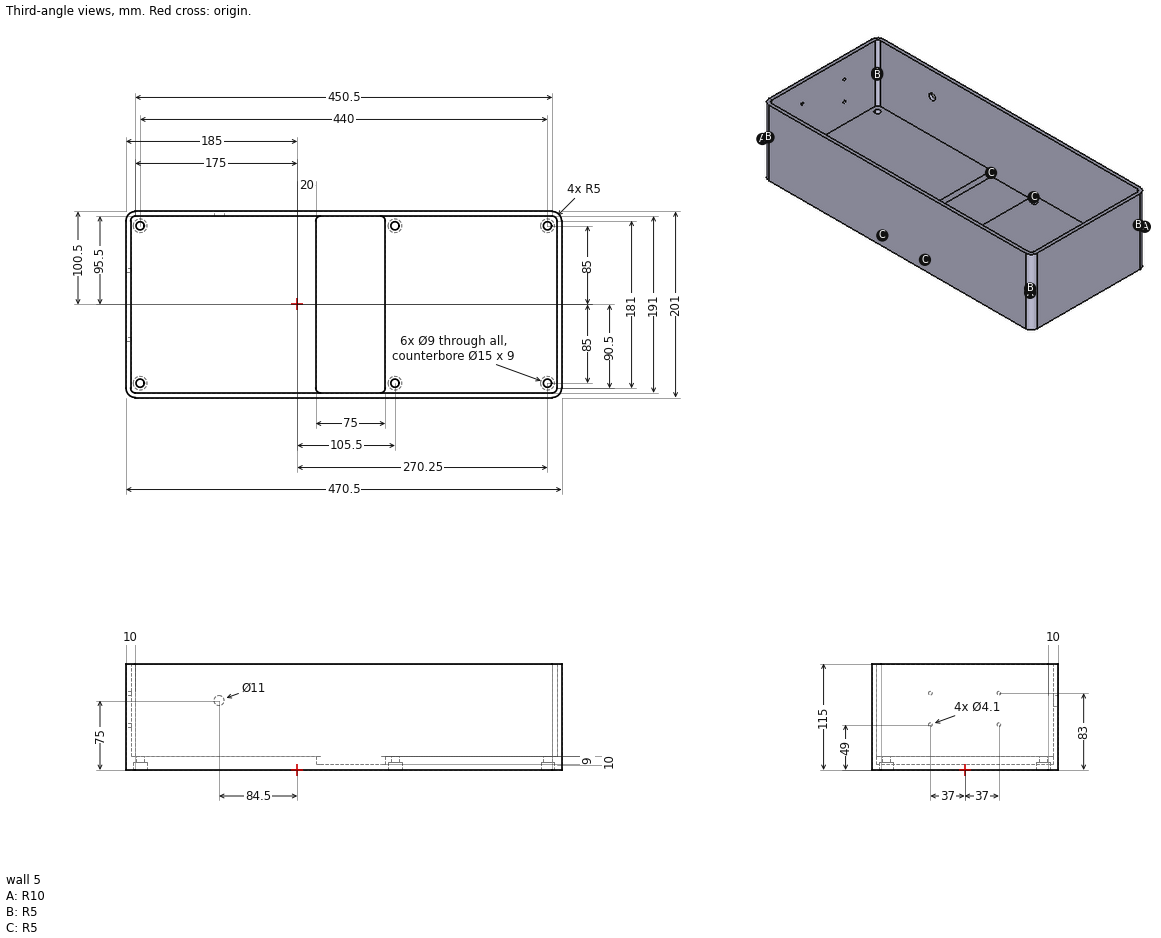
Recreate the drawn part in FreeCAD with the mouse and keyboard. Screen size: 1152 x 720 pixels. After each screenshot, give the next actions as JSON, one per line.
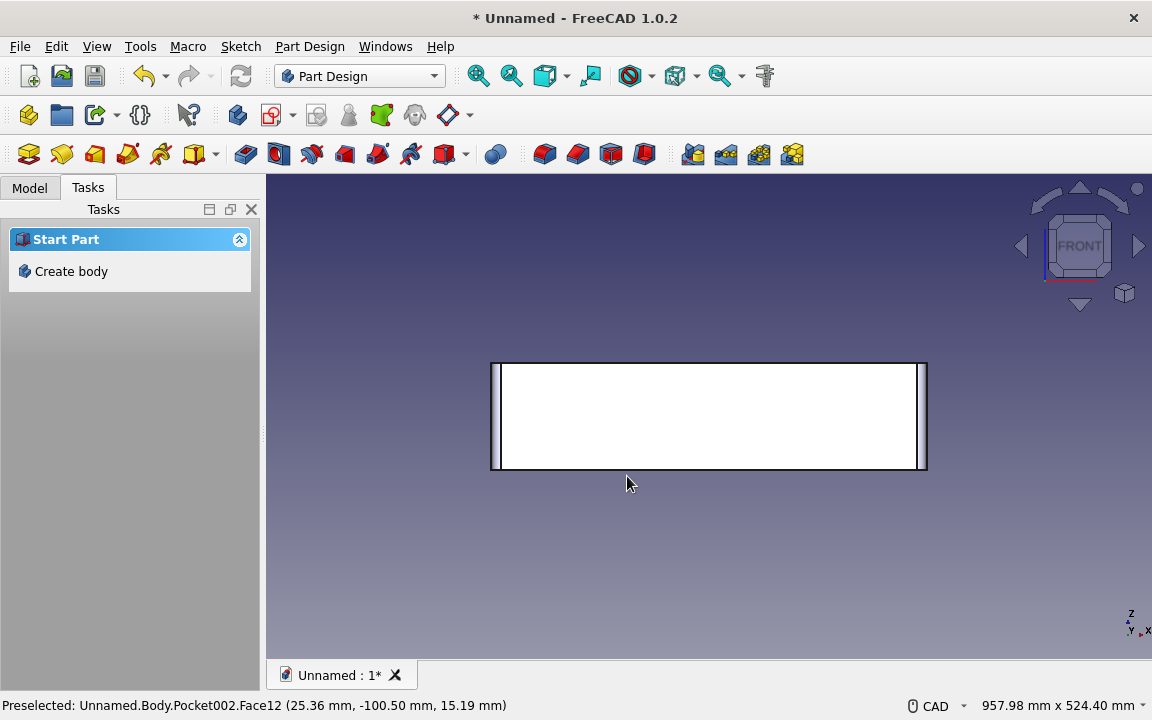
{"action": "scroll", "coordinate": [681, 459], "scroll_direction": "up", "scroll_amount": 8}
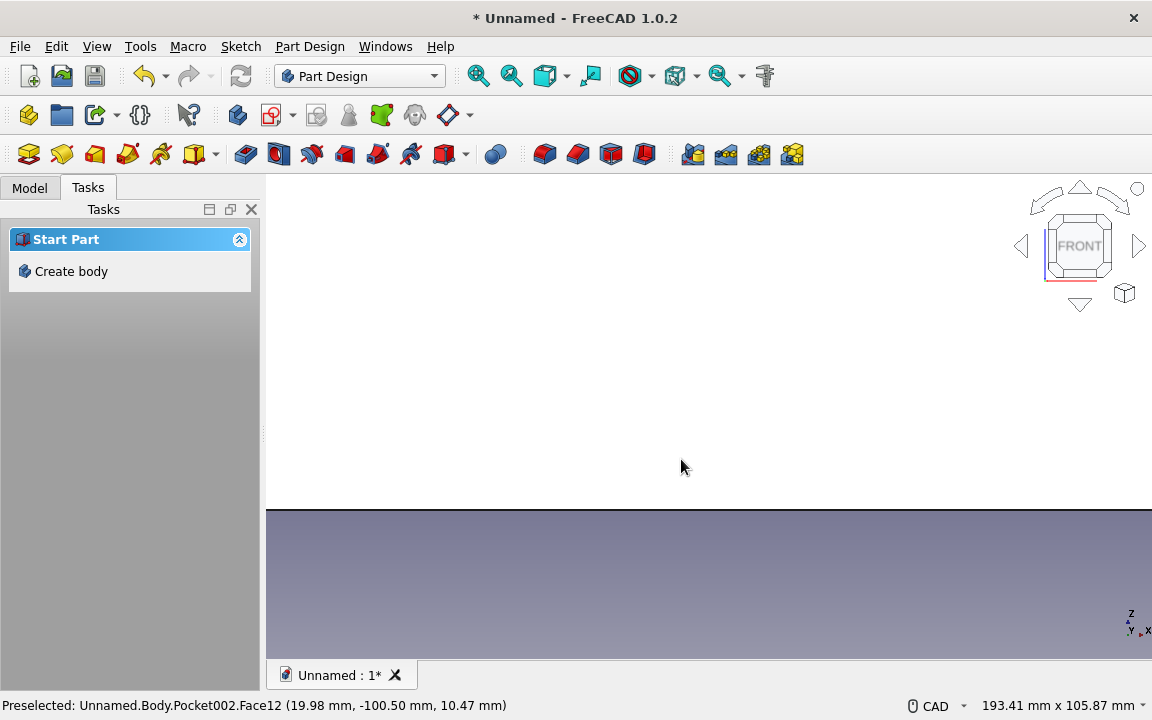
{"action": "key", "text": "v f"}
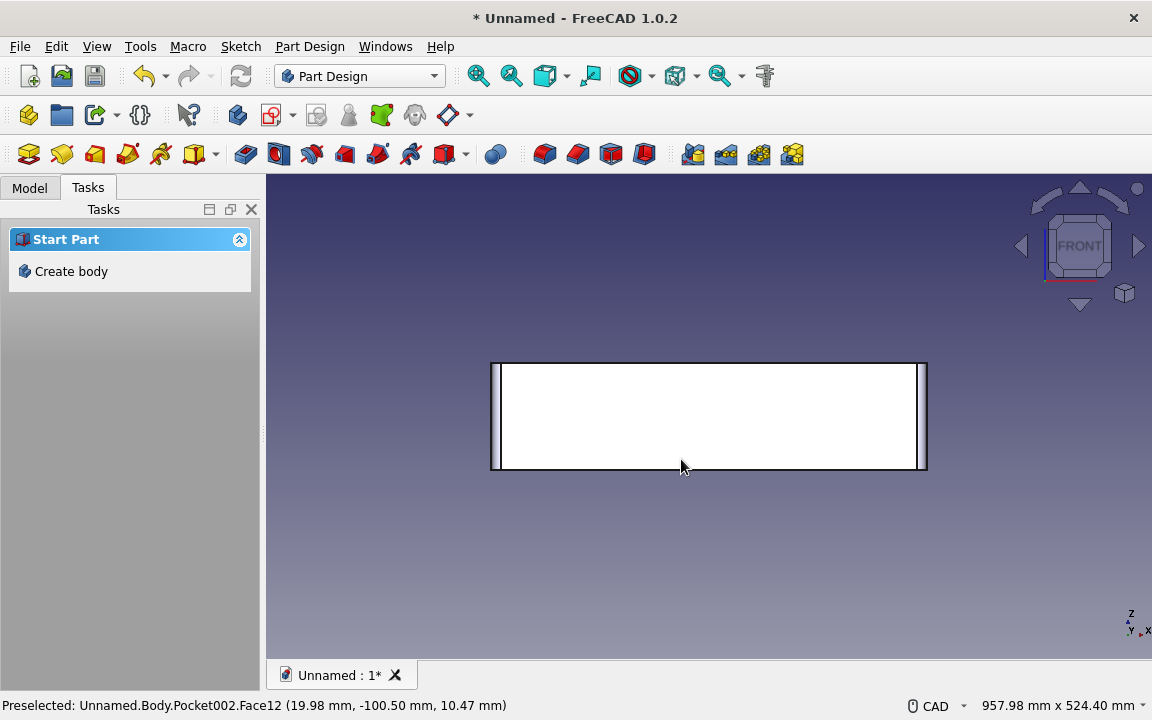
{"action": "key", "text": "3"}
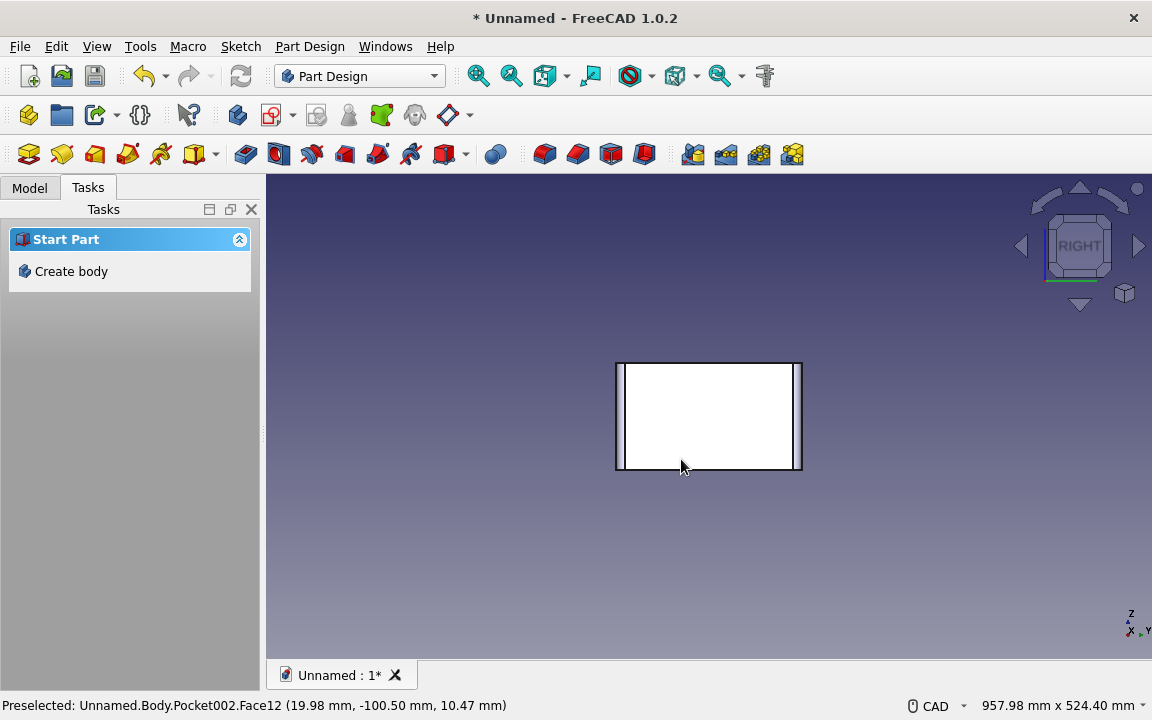
{"action": "key", "text": "v f"}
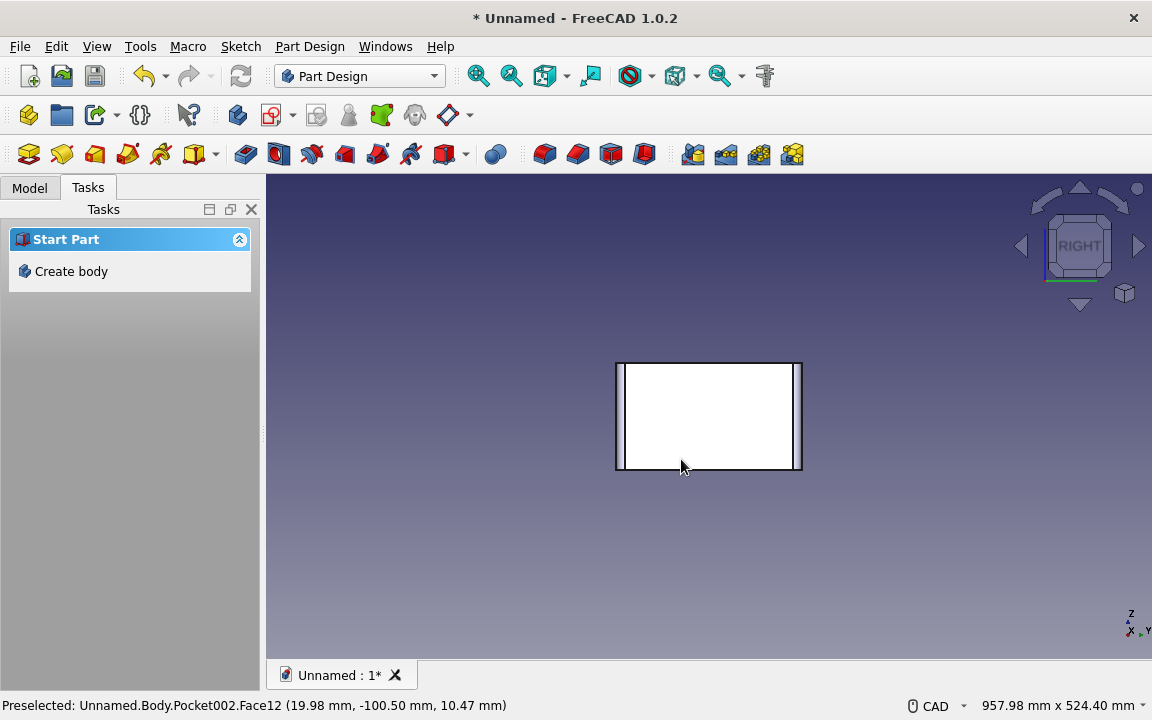
{"action": "scroll", "coordinate": [621, 459], "scroll_direction": "up", "scroll_amount": 8}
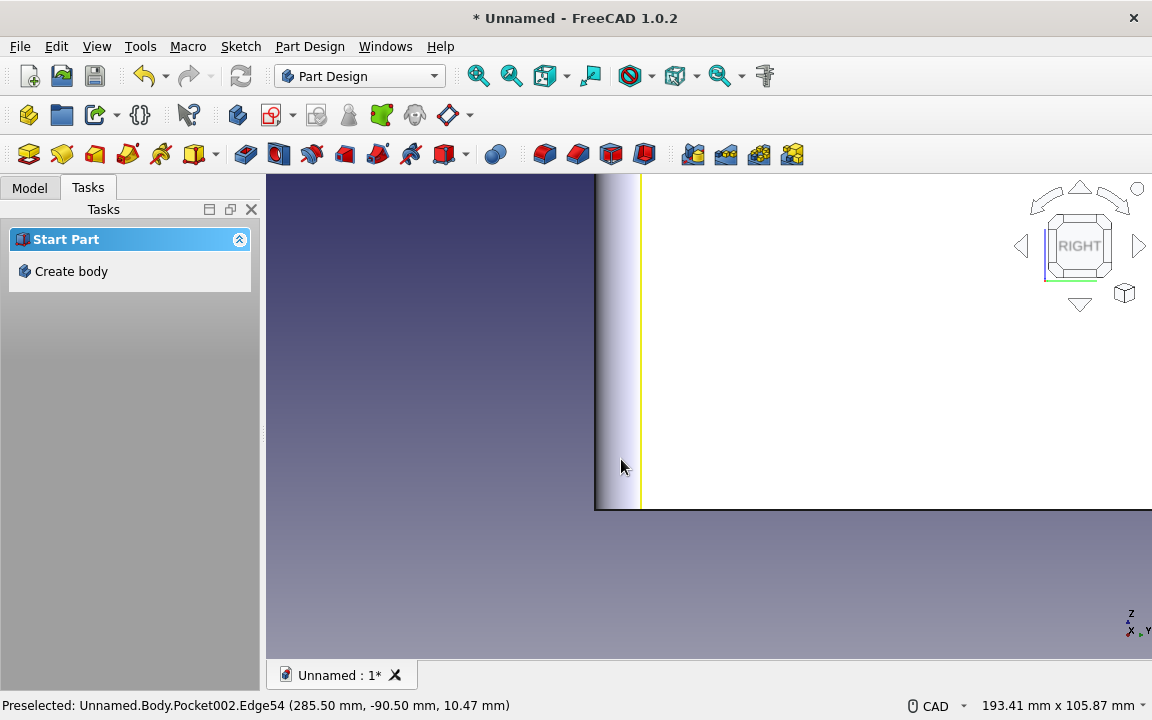
{"action": "key", "text": "v f"}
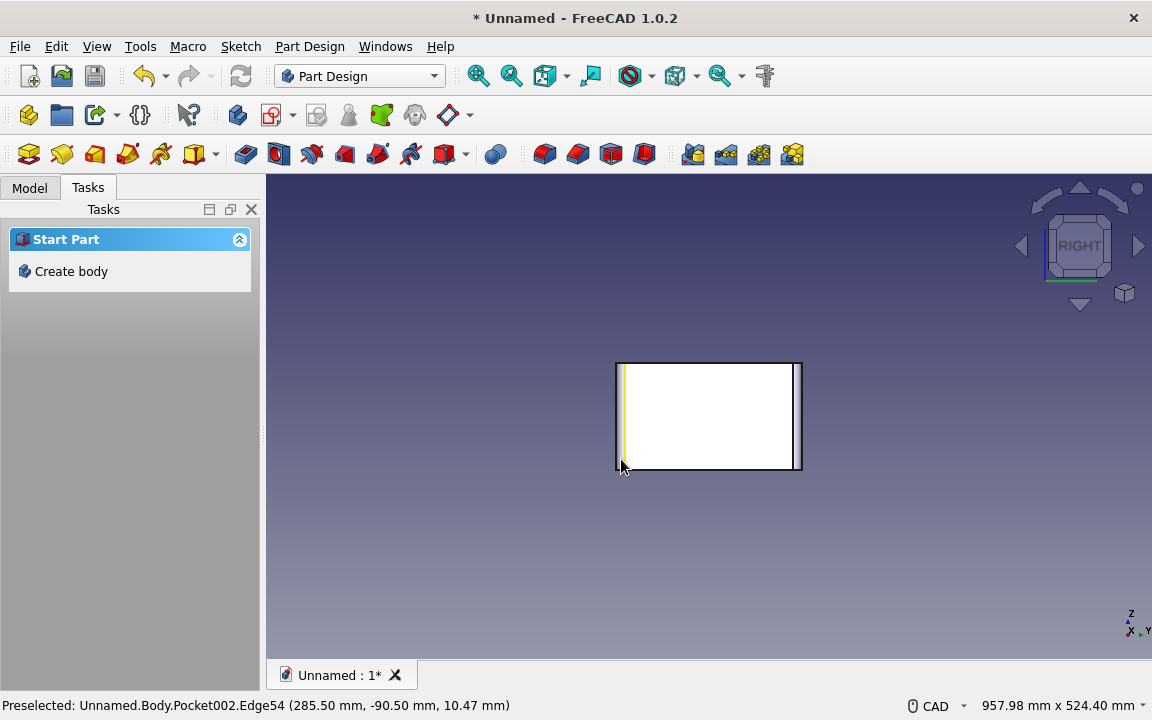
{"action": "key", "text": "5"}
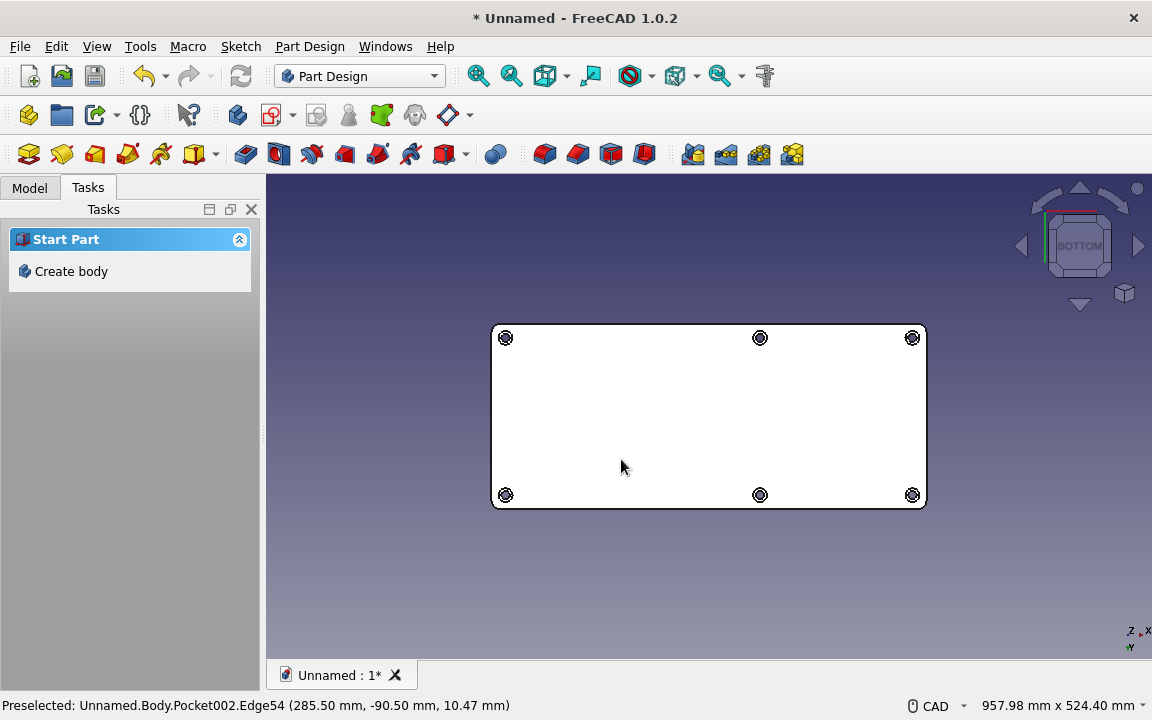
{"action": "scroll", "coordinate": [681, 327], "scroll_direction": "up", "scroll_amount": 8}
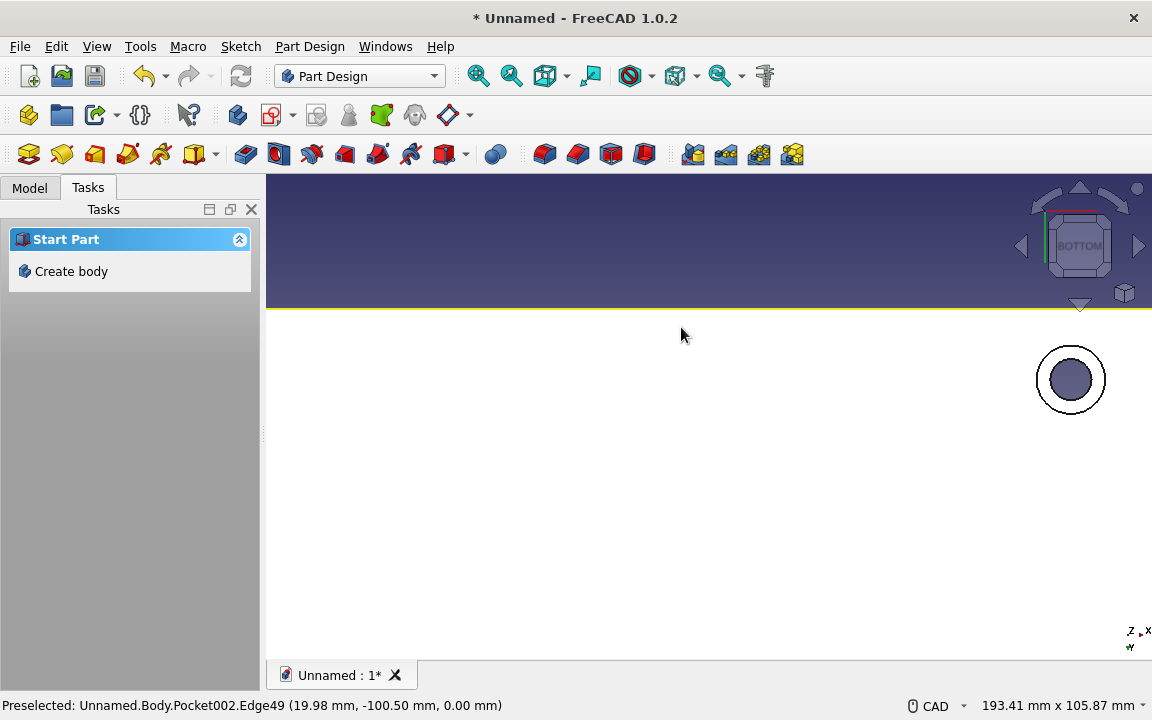
{"action": "left_click", "coordinate": [479, 76]}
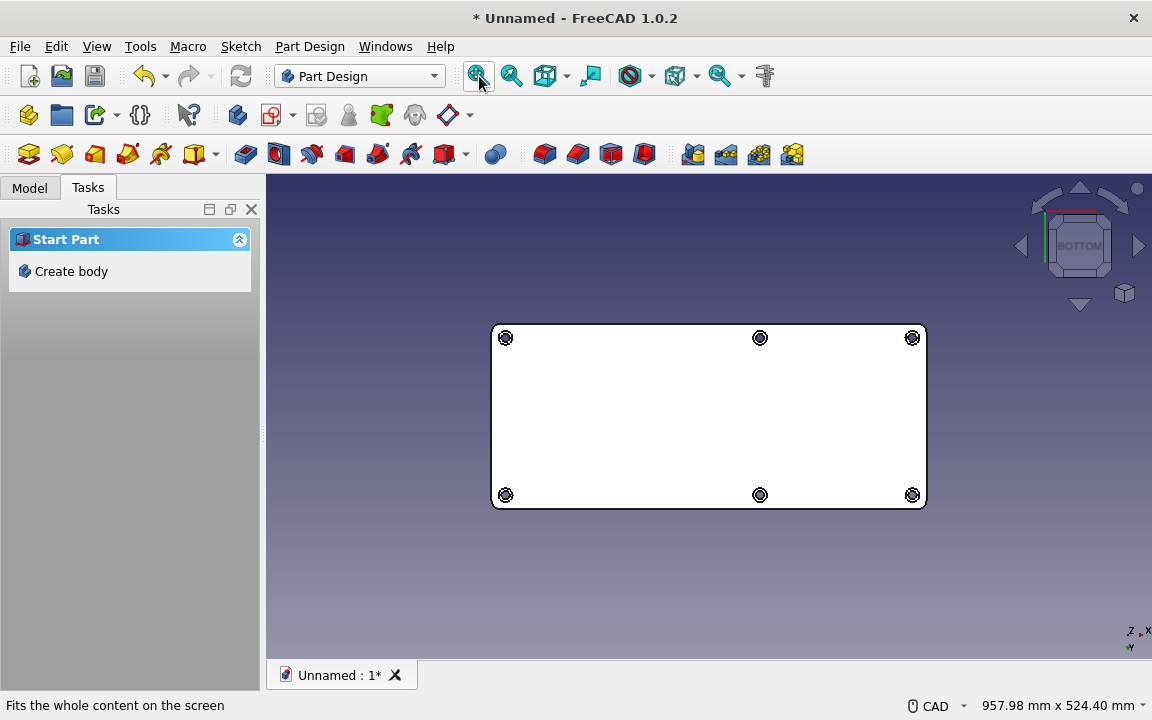
{"action": "key", "text": "4"}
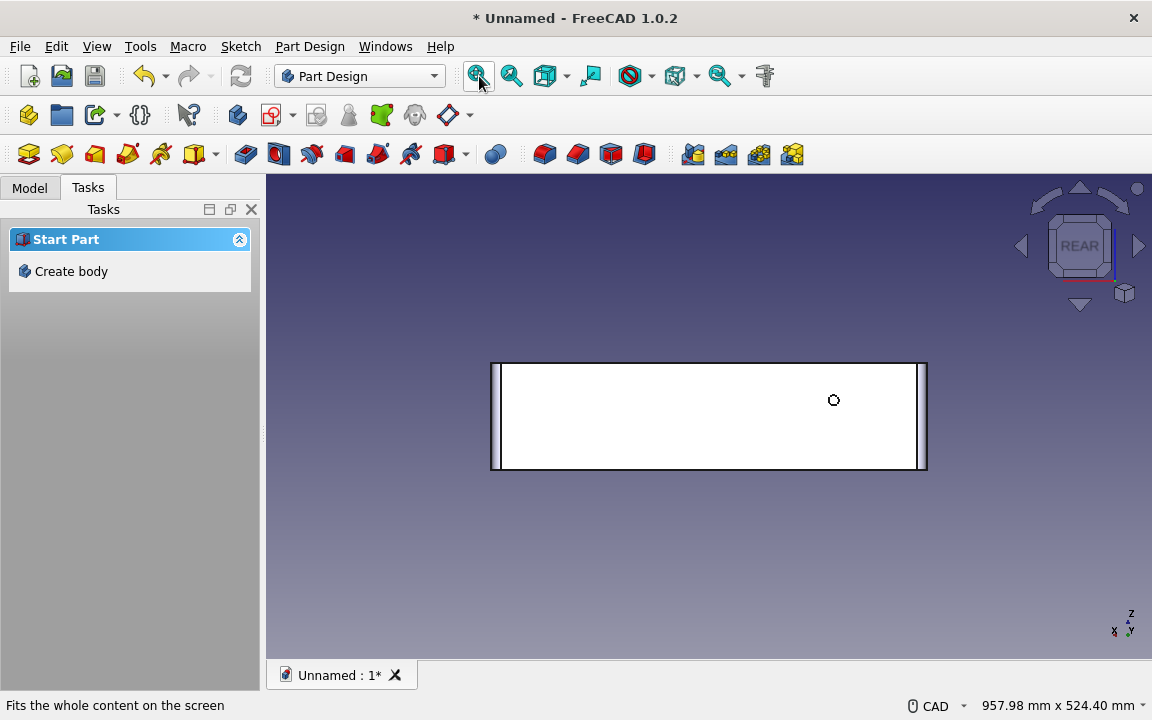
{"action": "scroll", "coordinate": [737, 459], "scroll_direction": "up", "scroll_amount": 8}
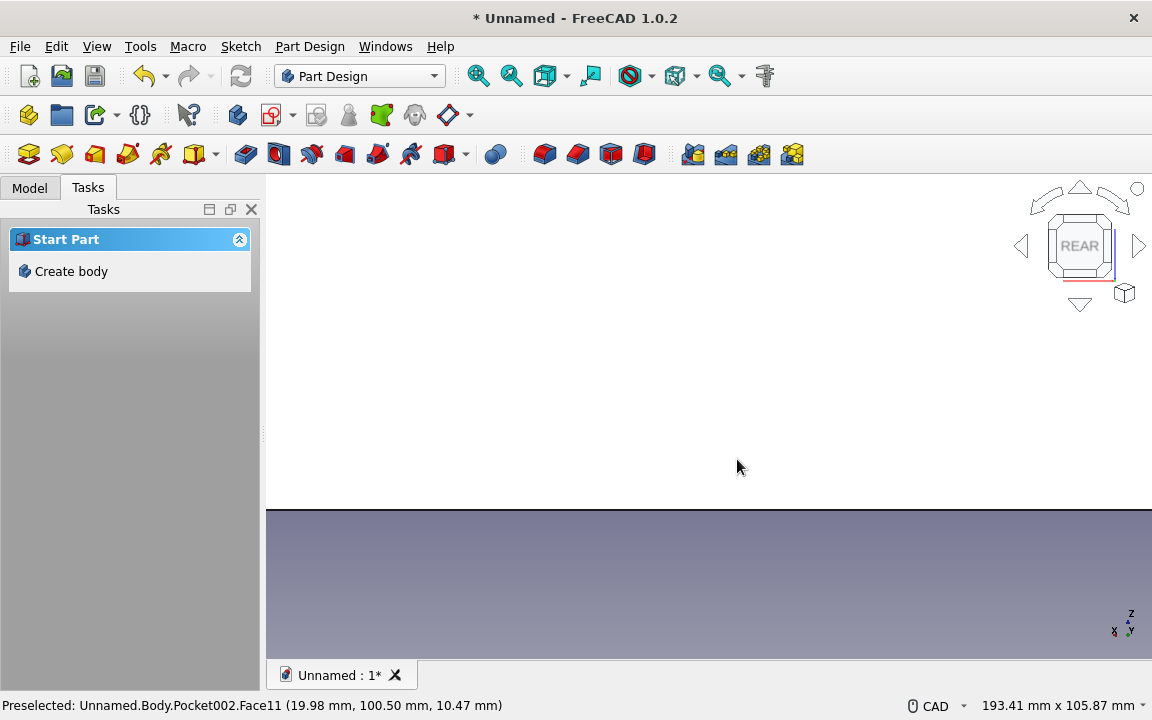
{"action": "key", "text": "v f"}